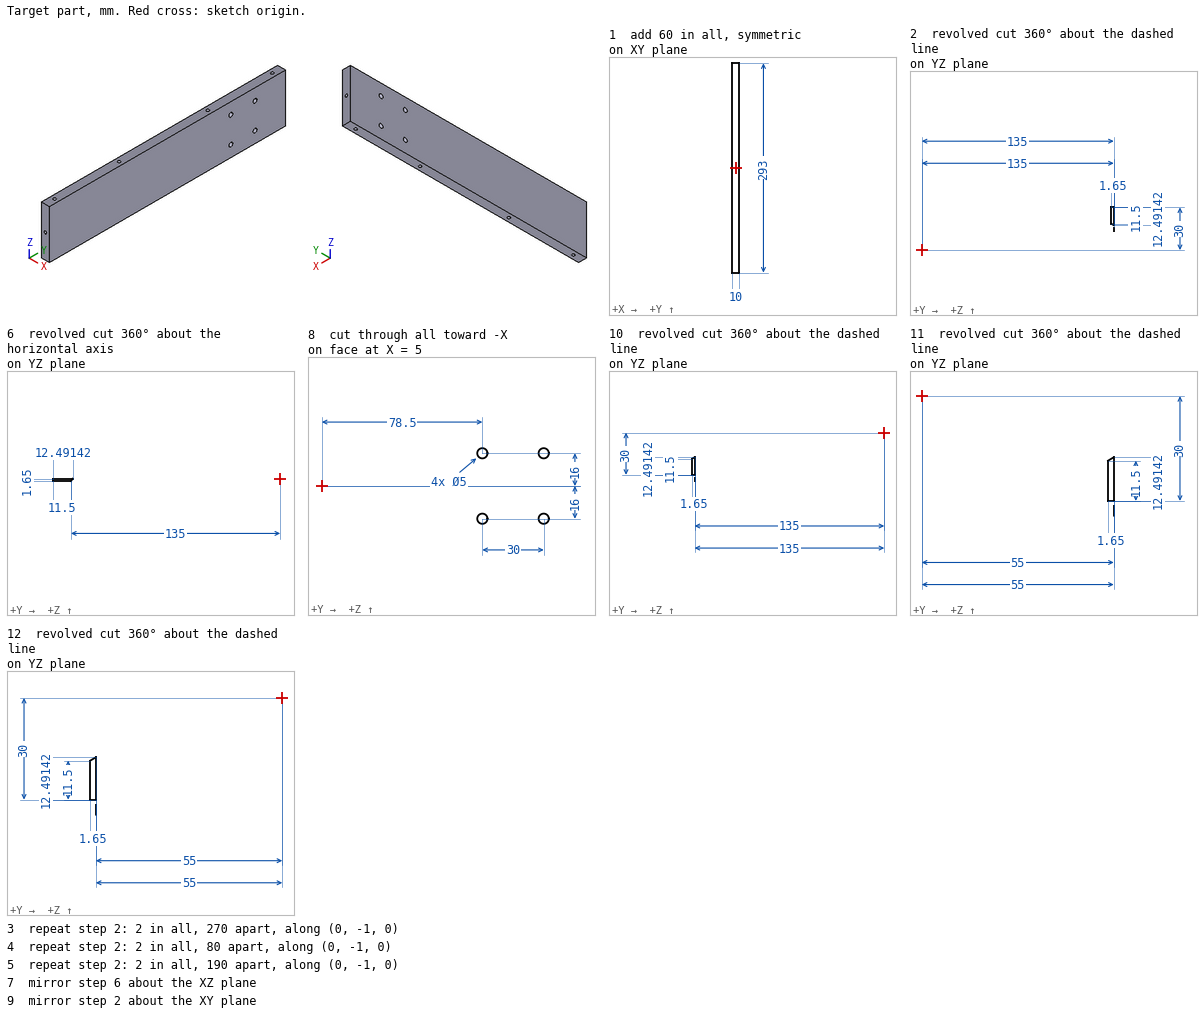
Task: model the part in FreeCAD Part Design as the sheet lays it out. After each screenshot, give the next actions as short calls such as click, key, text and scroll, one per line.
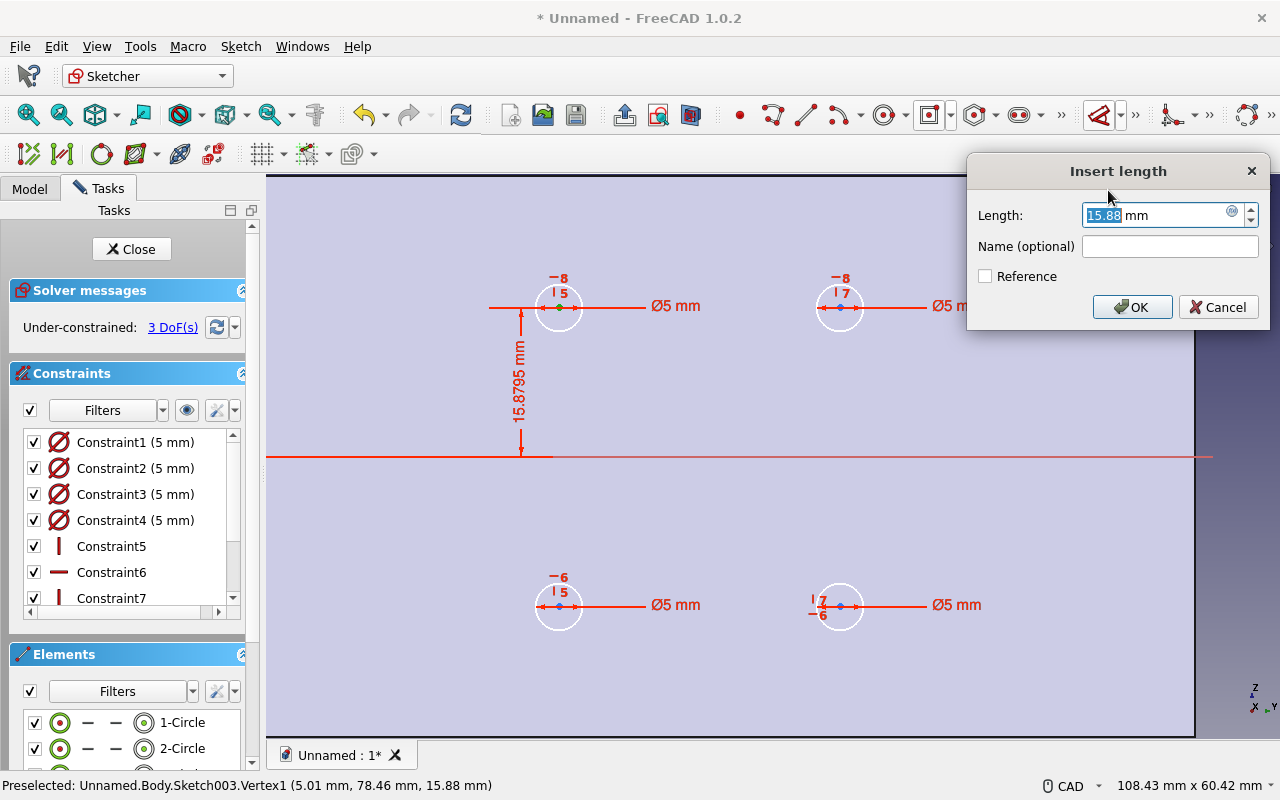
text(16)
key(Return)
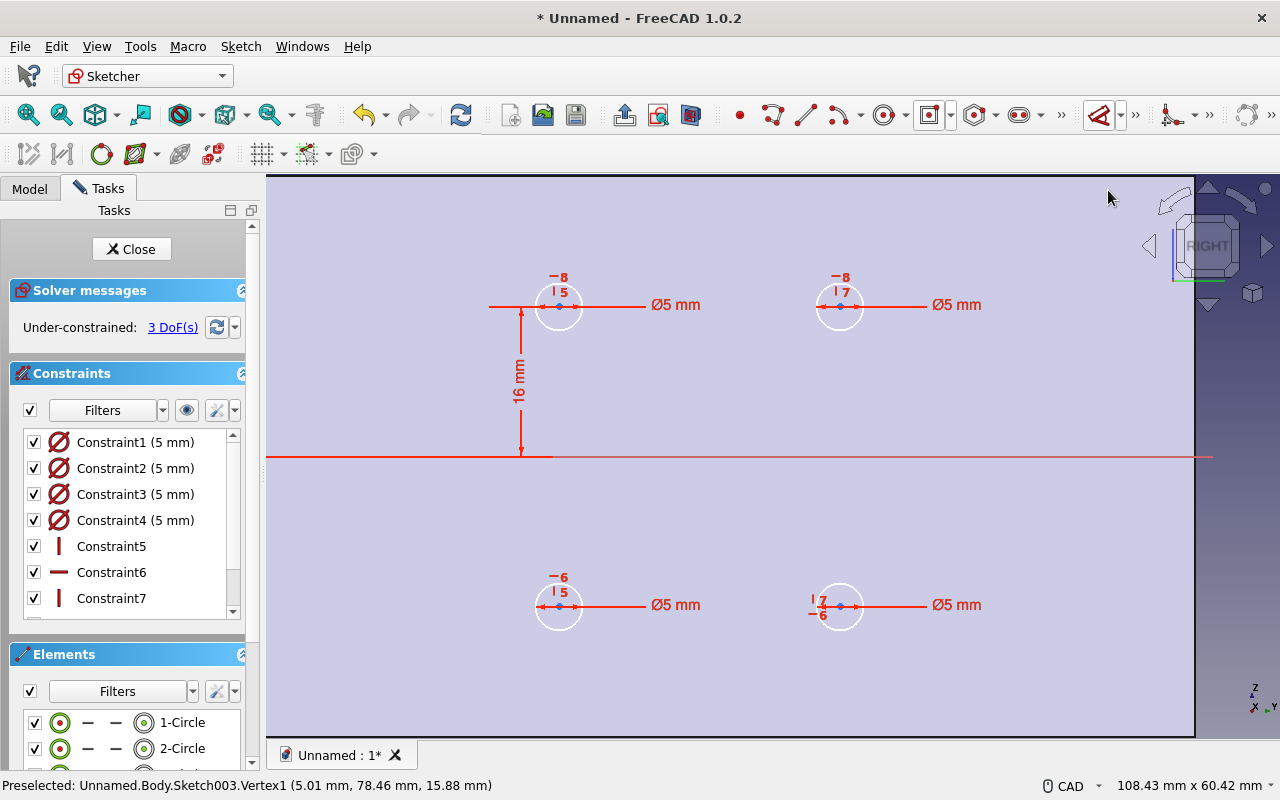
click(559, 607)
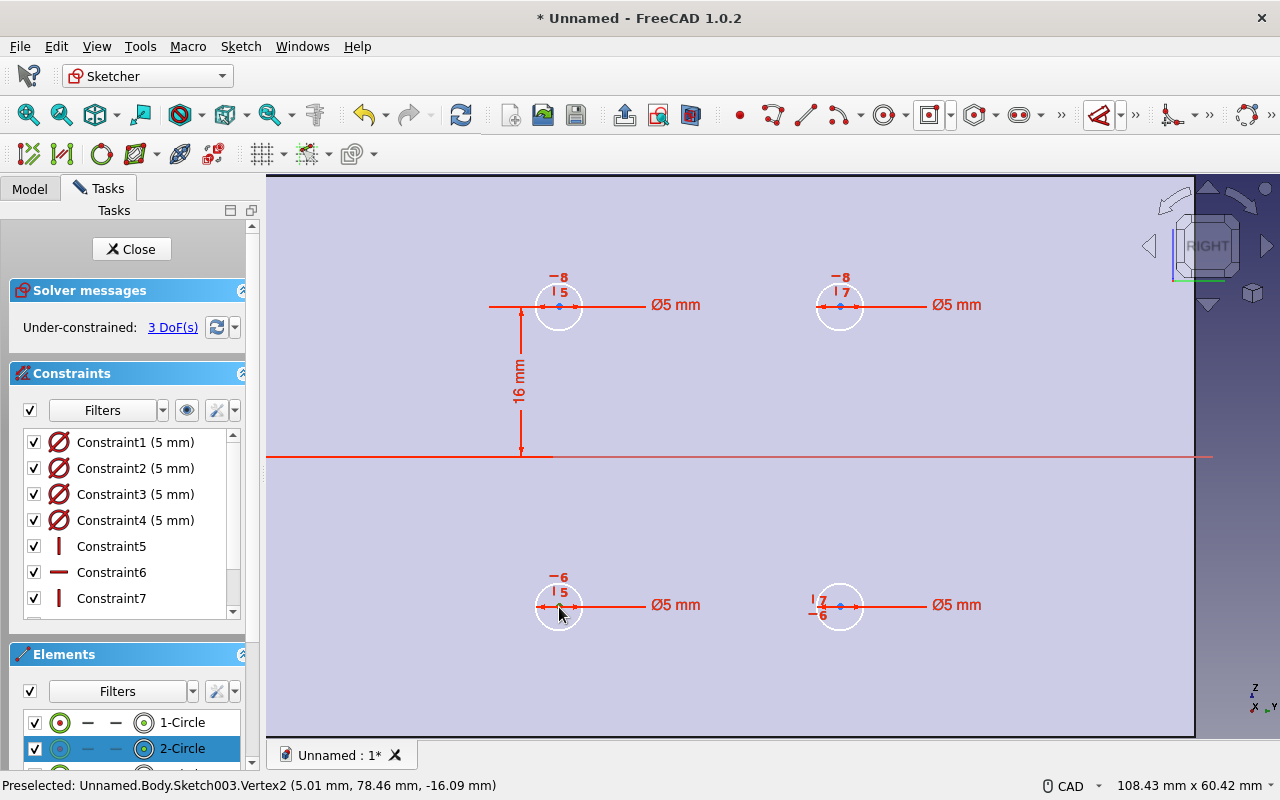
click(1120, 116)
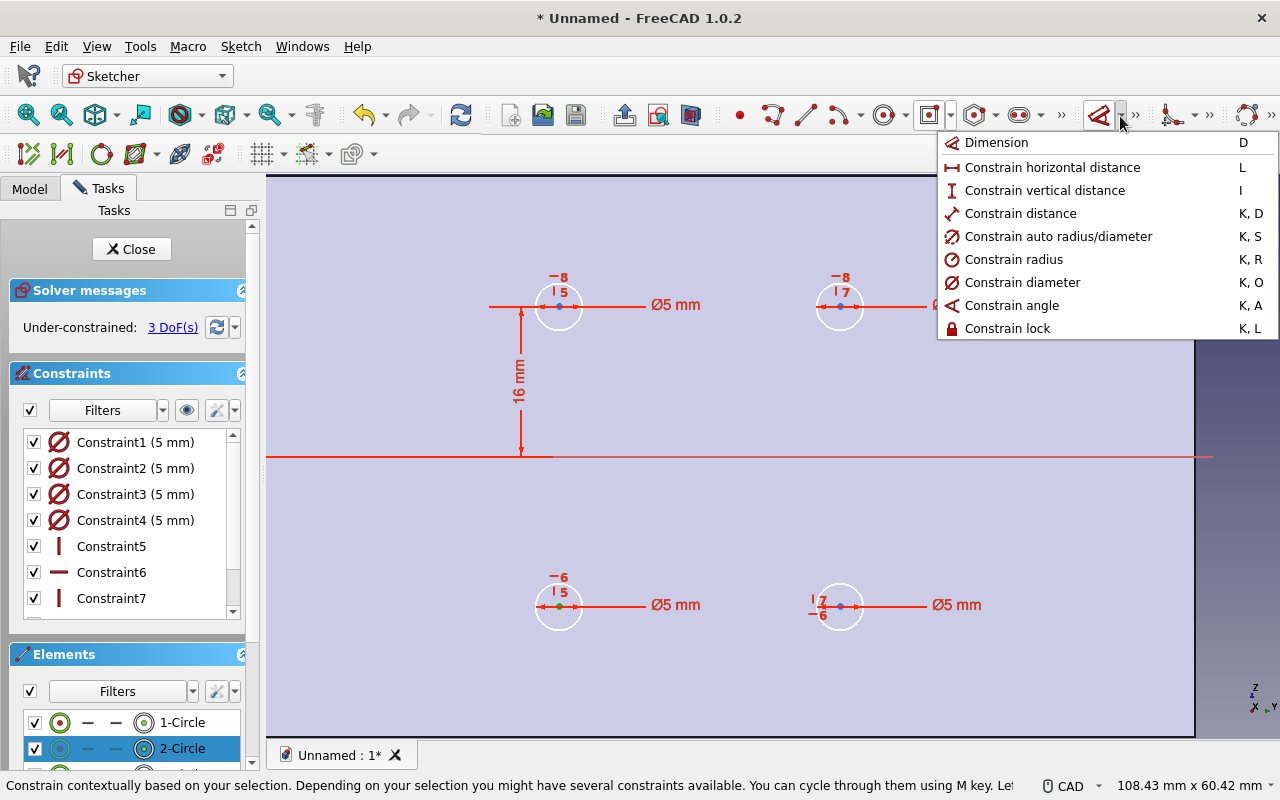
click(1108, 190)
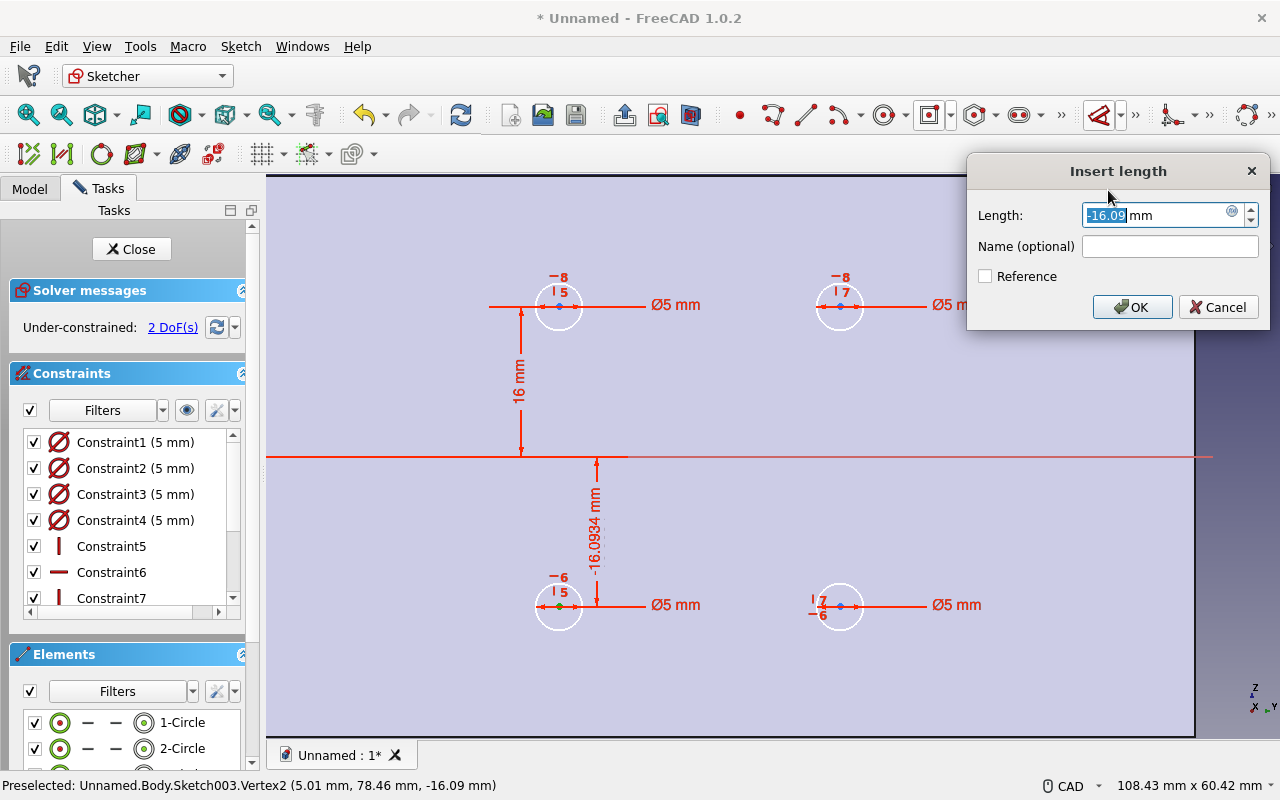
text(-16)
key(Return)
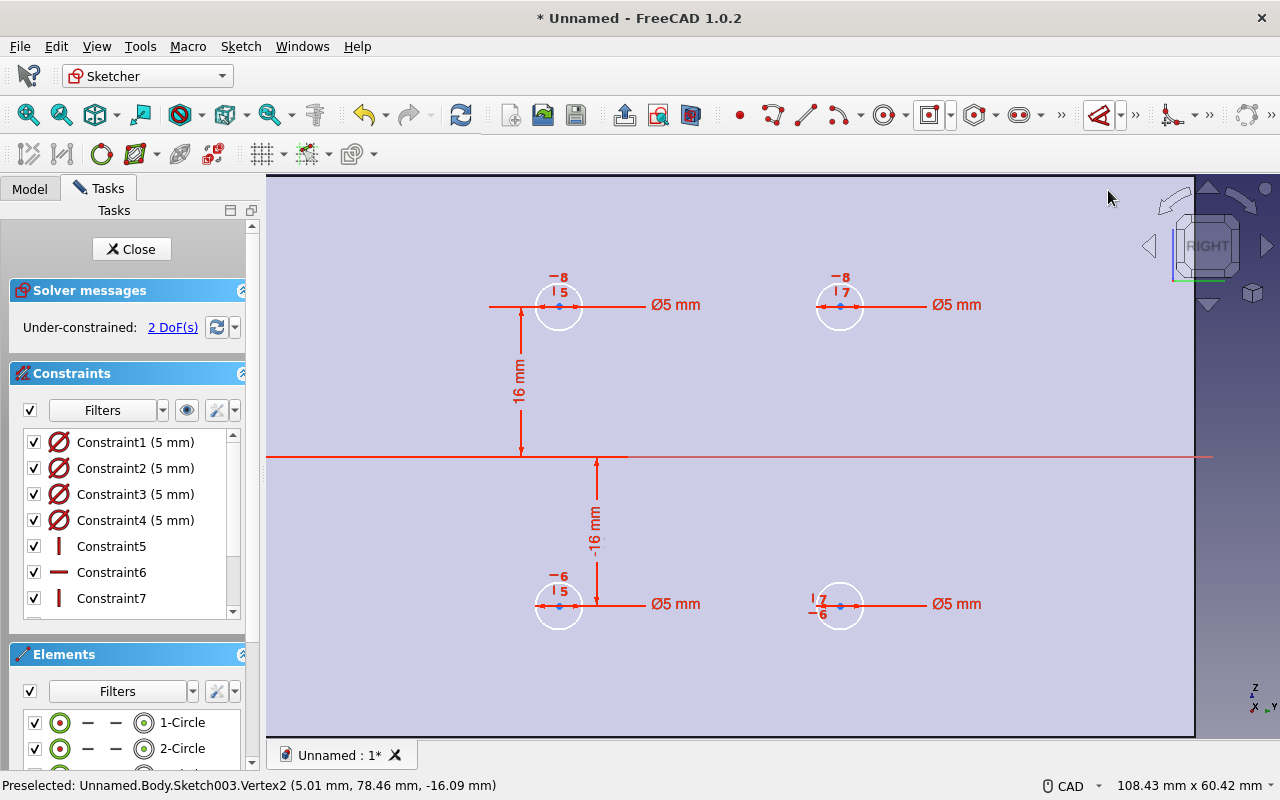
click(559, 606)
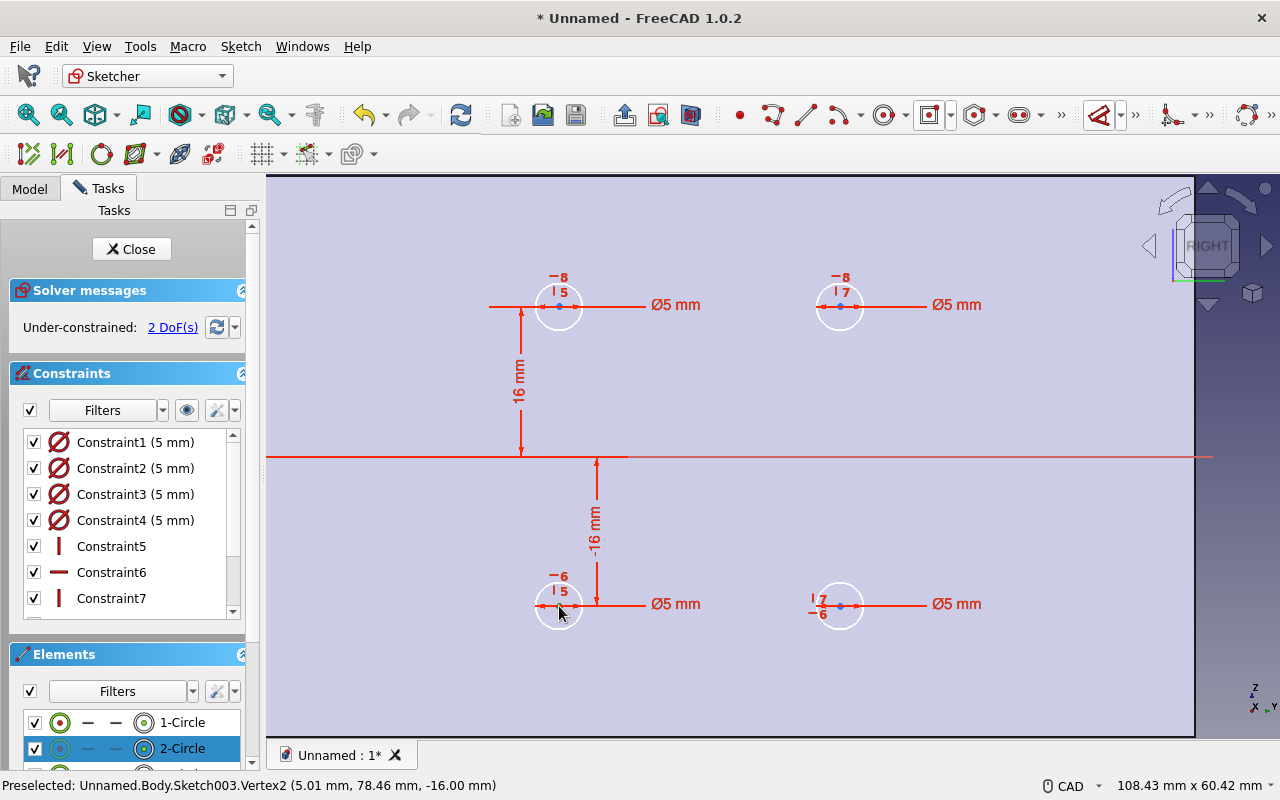
click(840, 606)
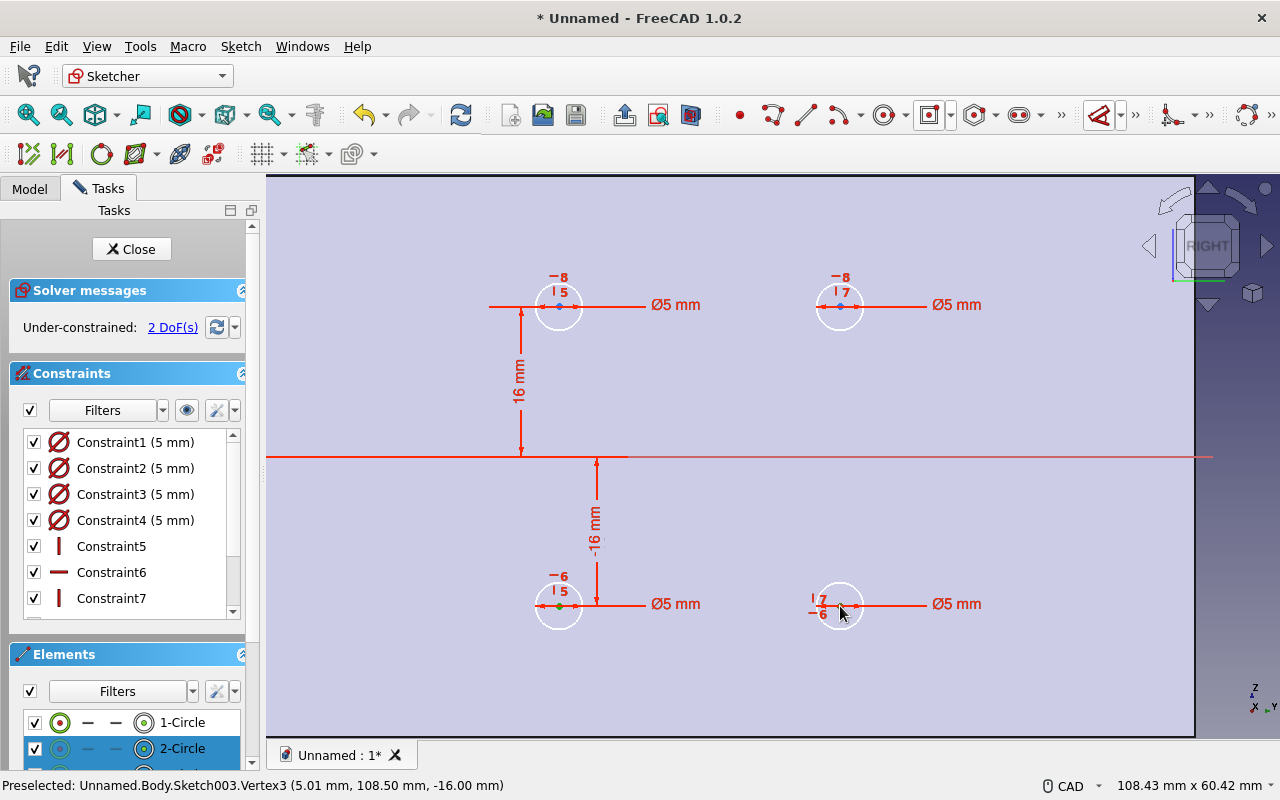
click(1120, 116)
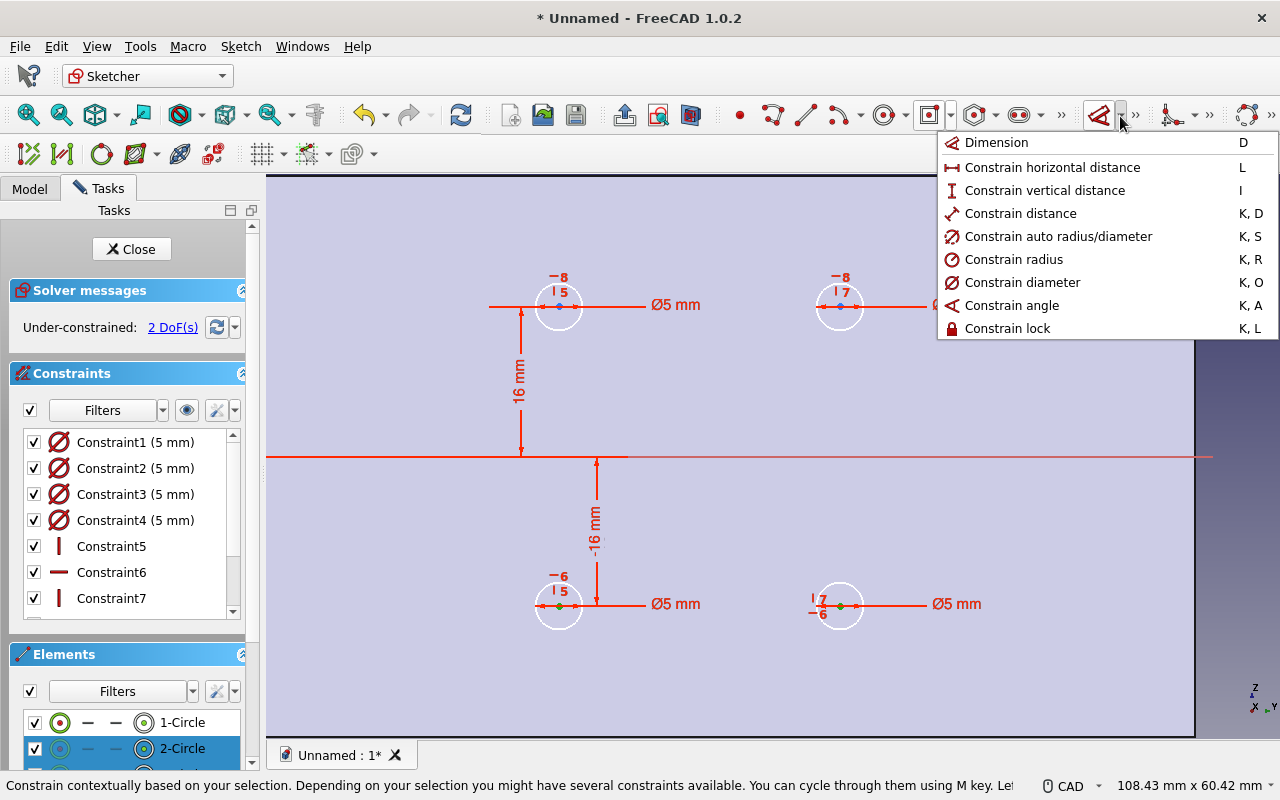
click(1108, 168)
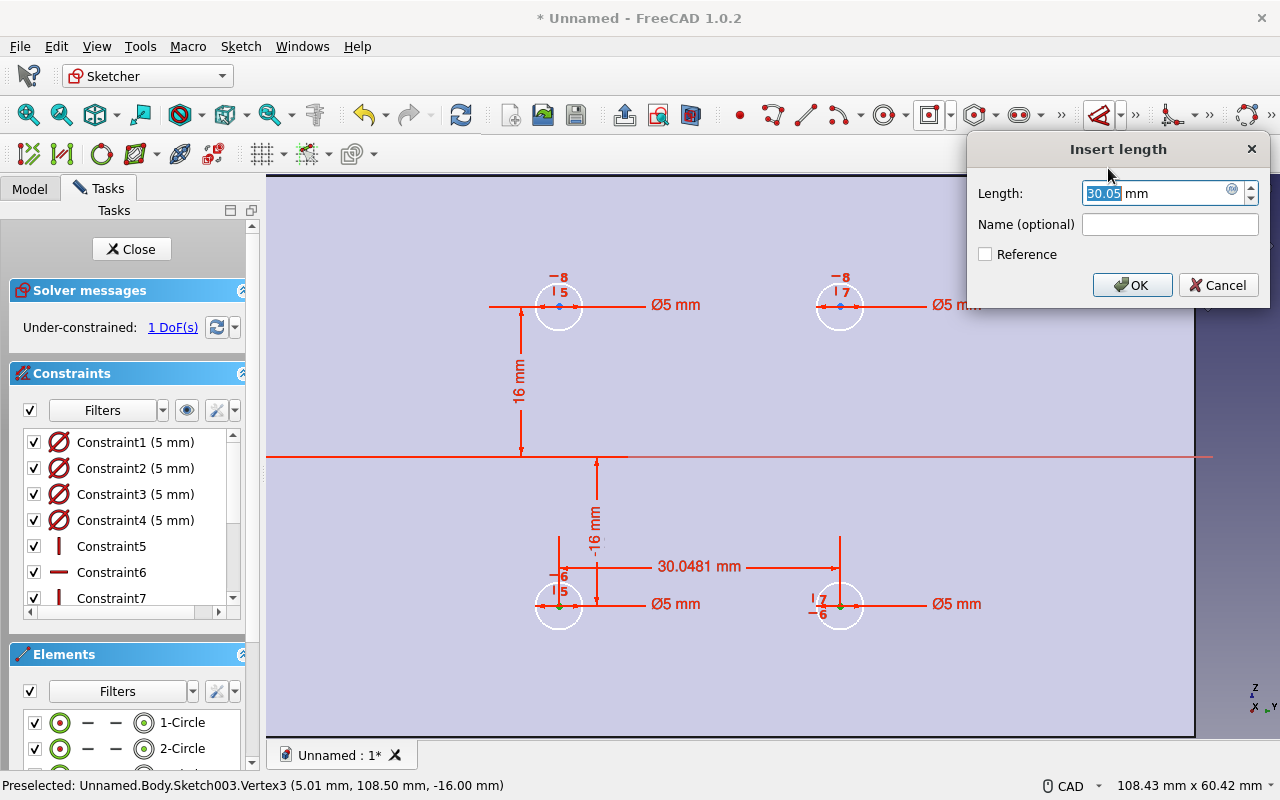
text(30)
key(Return)